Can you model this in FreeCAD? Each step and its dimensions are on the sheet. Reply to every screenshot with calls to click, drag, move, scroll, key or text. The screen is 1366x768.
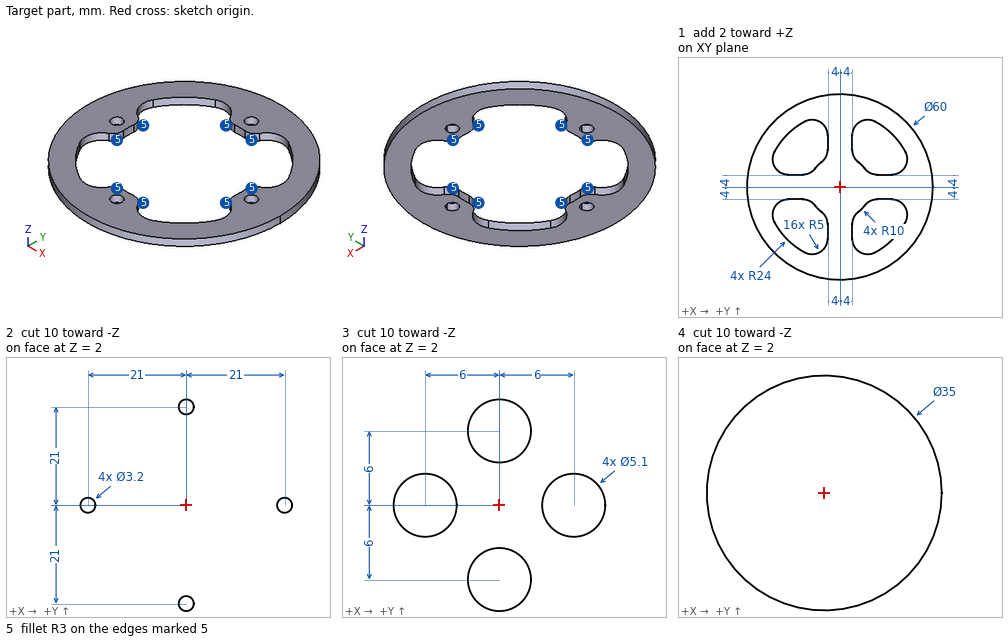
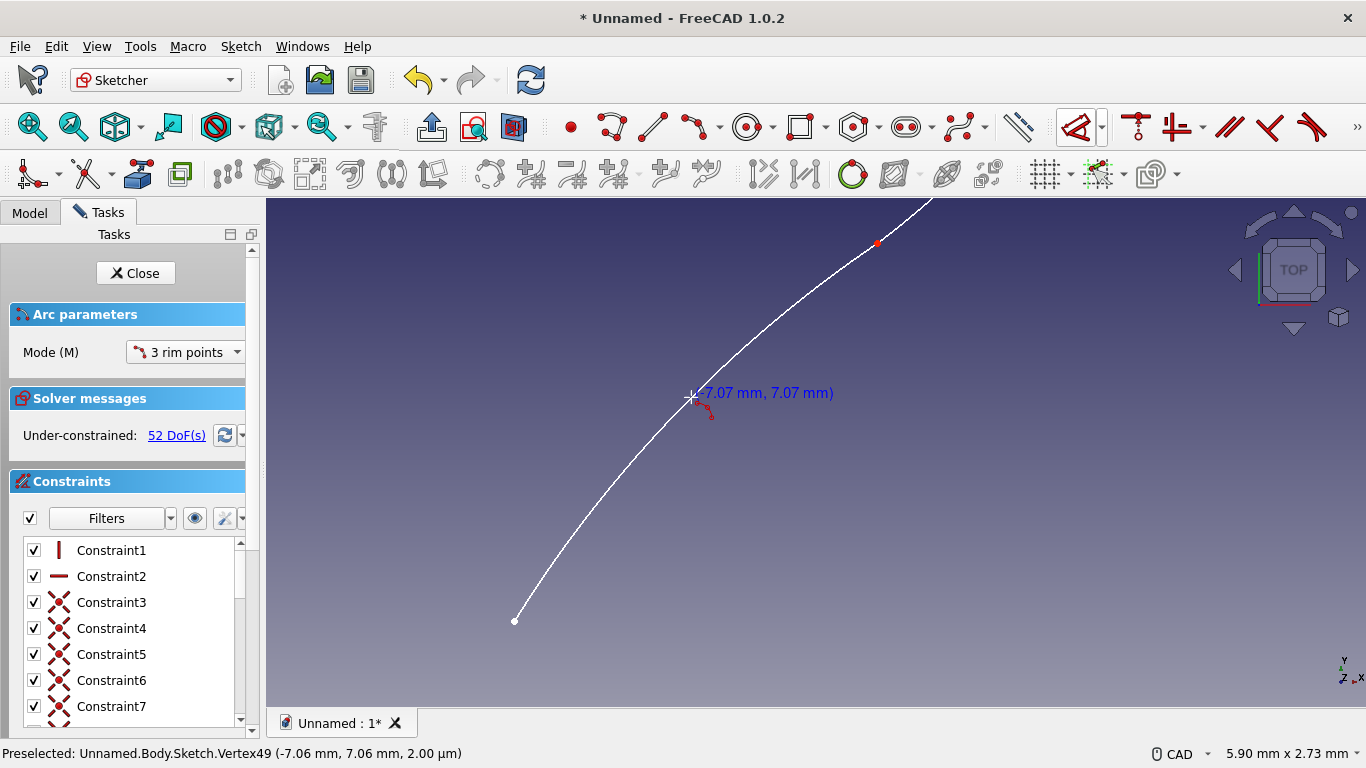
scroll(704, 409, down, 17)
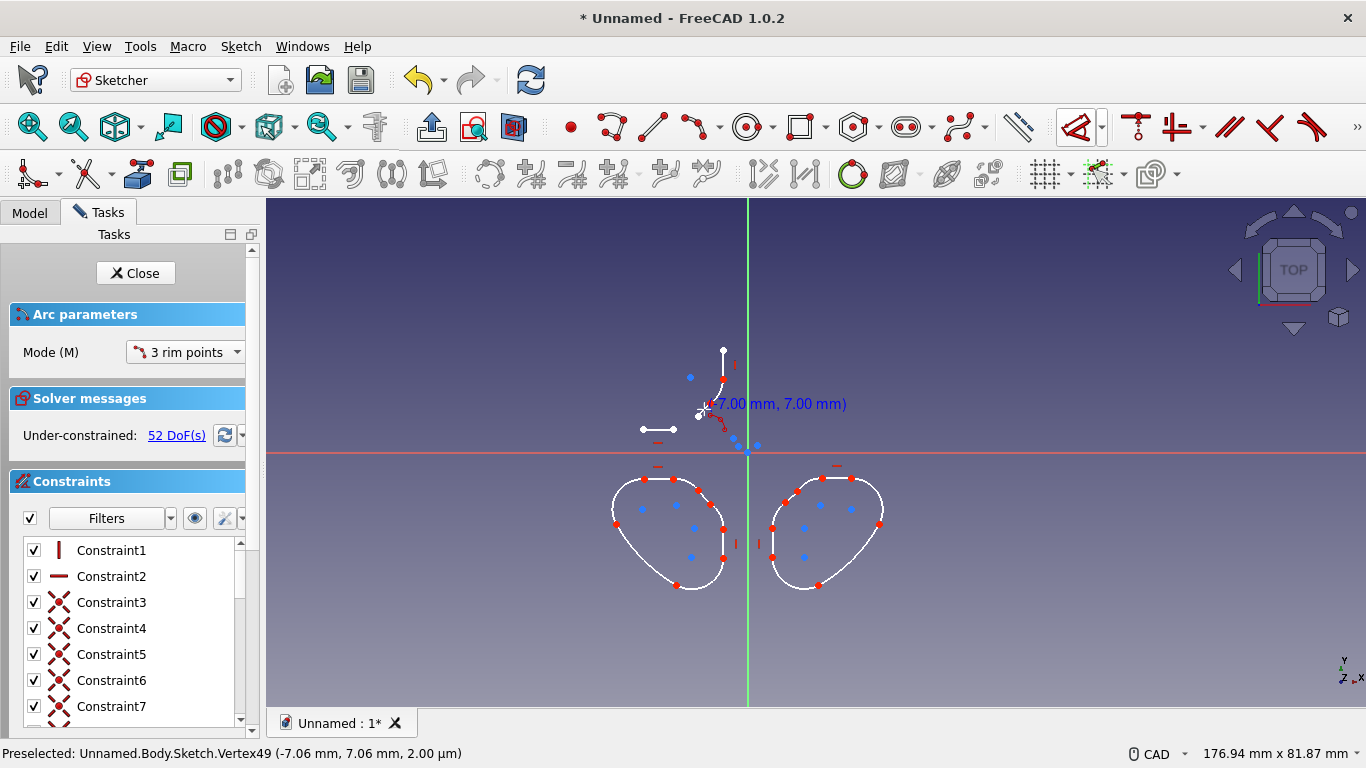
click(698, 416)
click(673, 430)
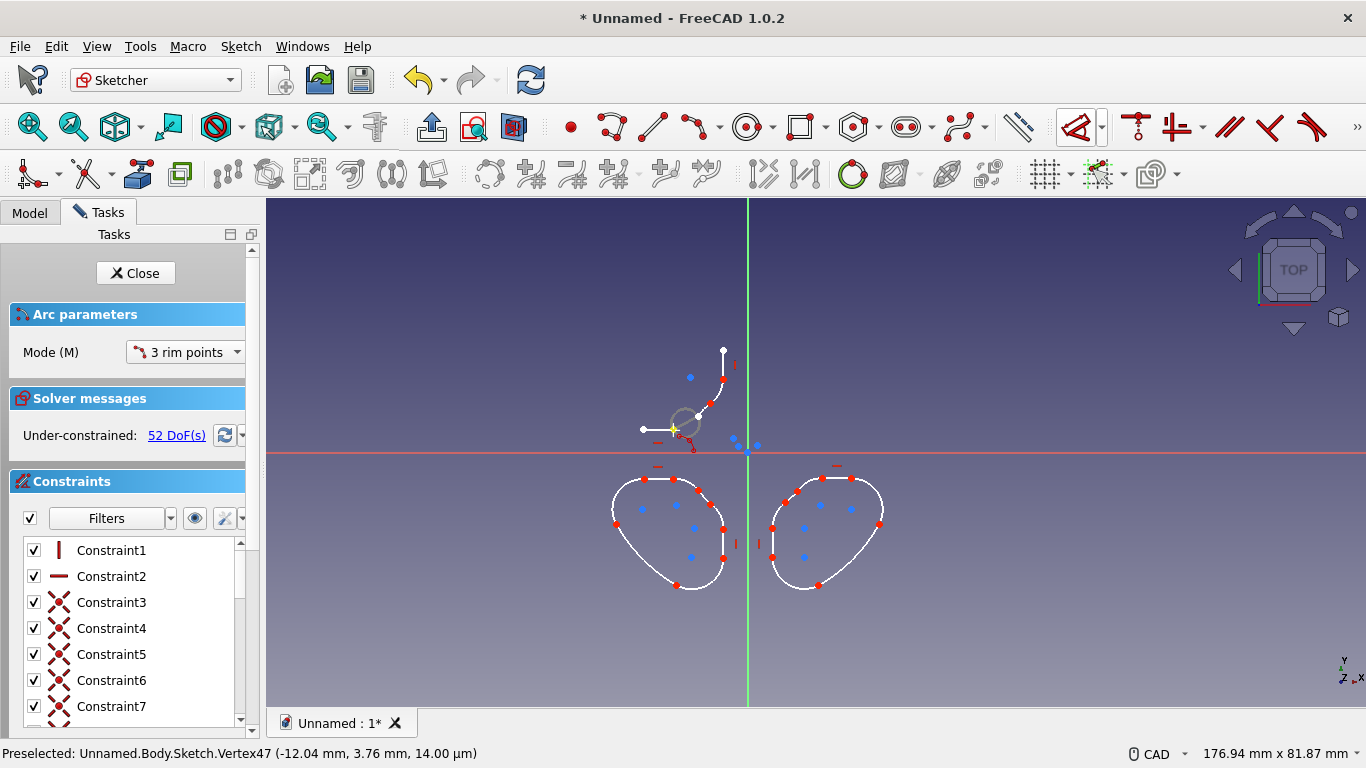
scroll(687, 425, up, 8)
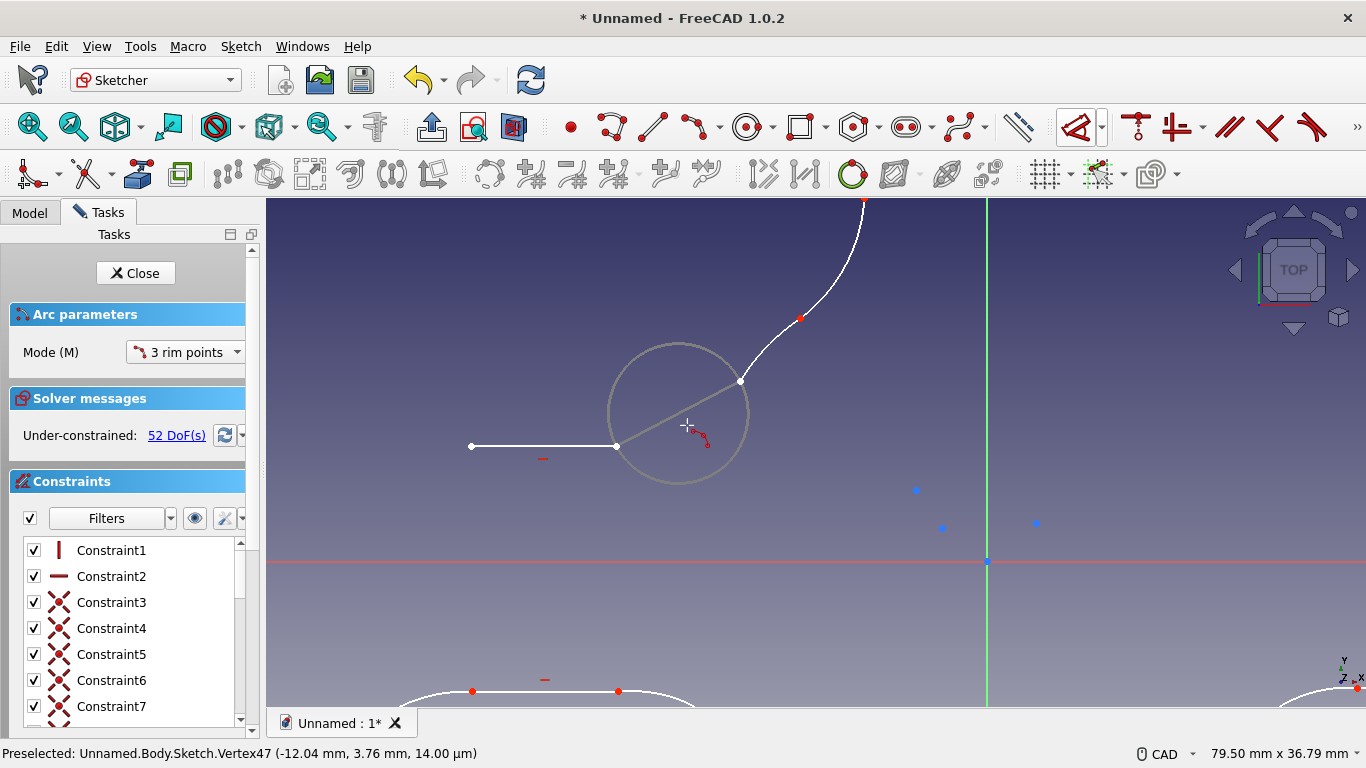
click(686, 422)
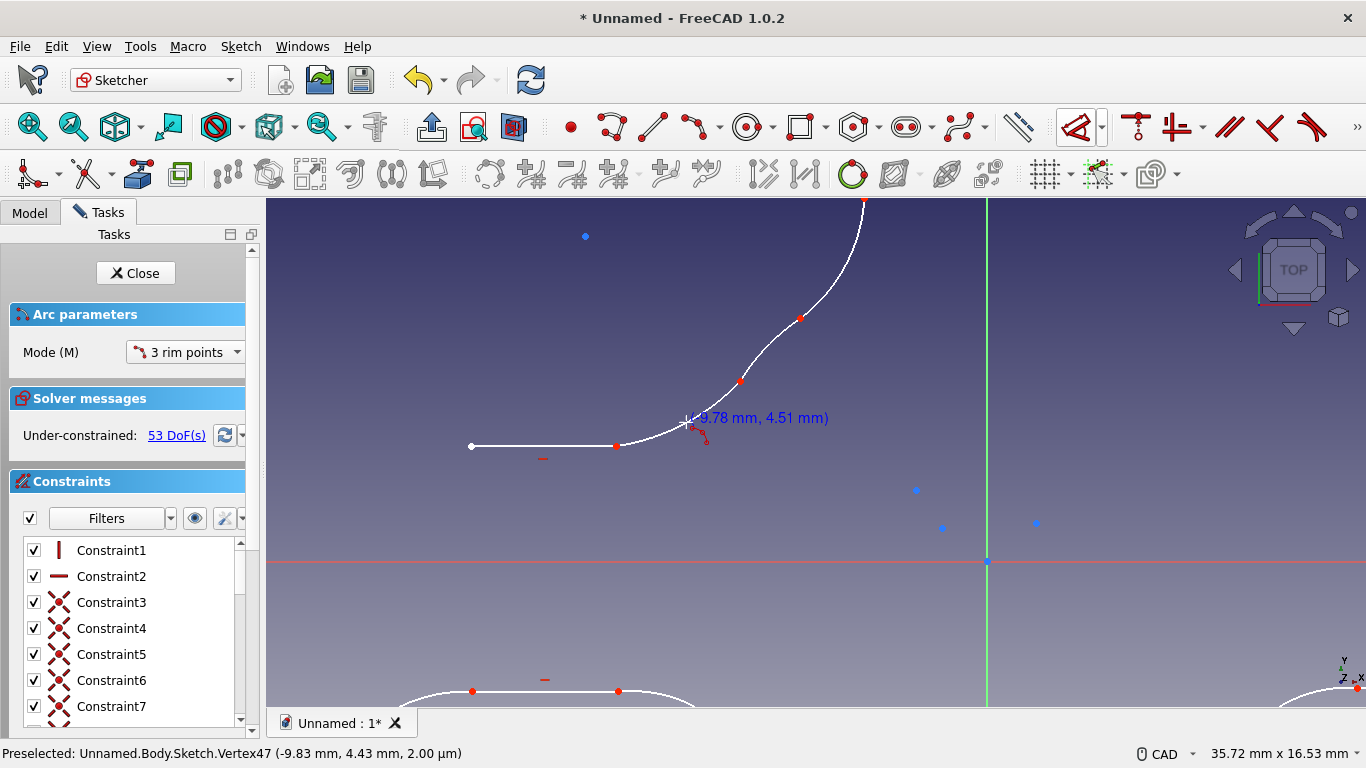
scroll(700, 431, down, 9)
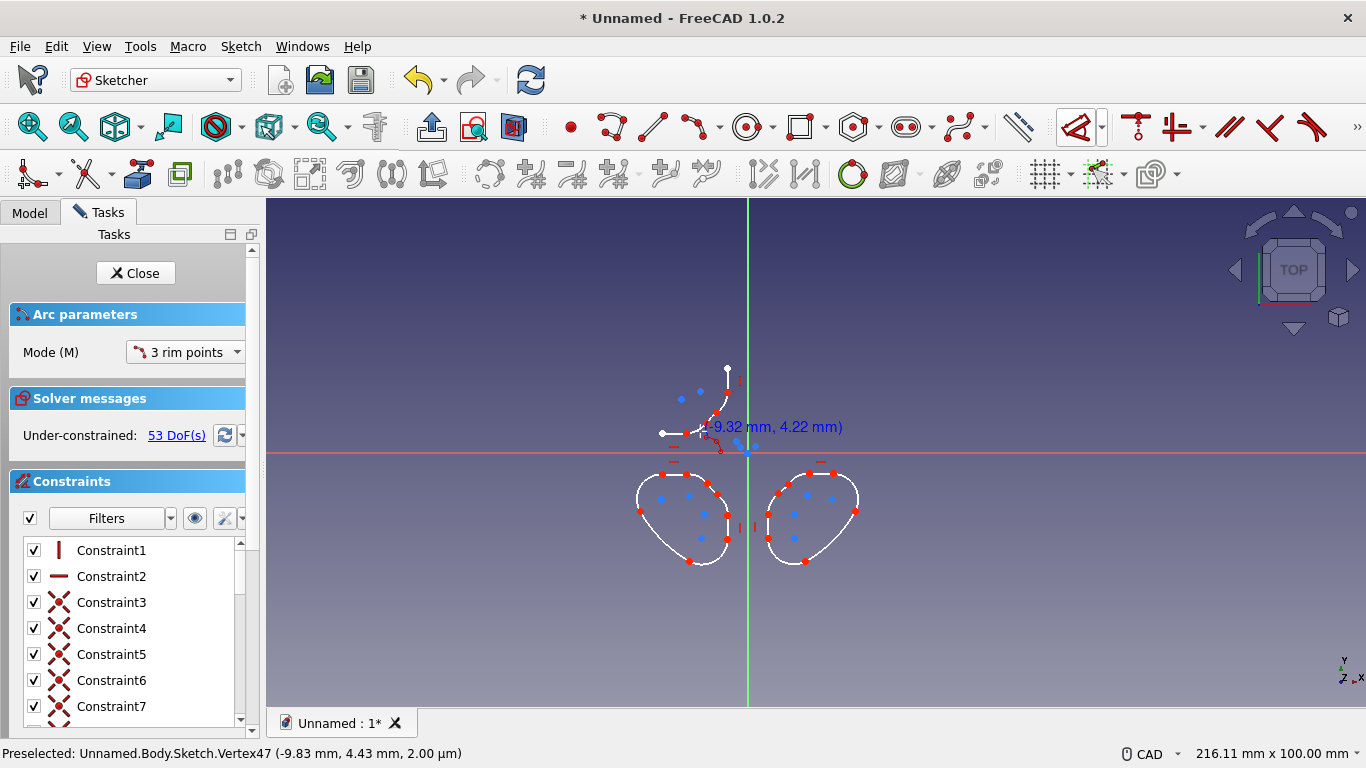
scroll(663, 433, up, 2)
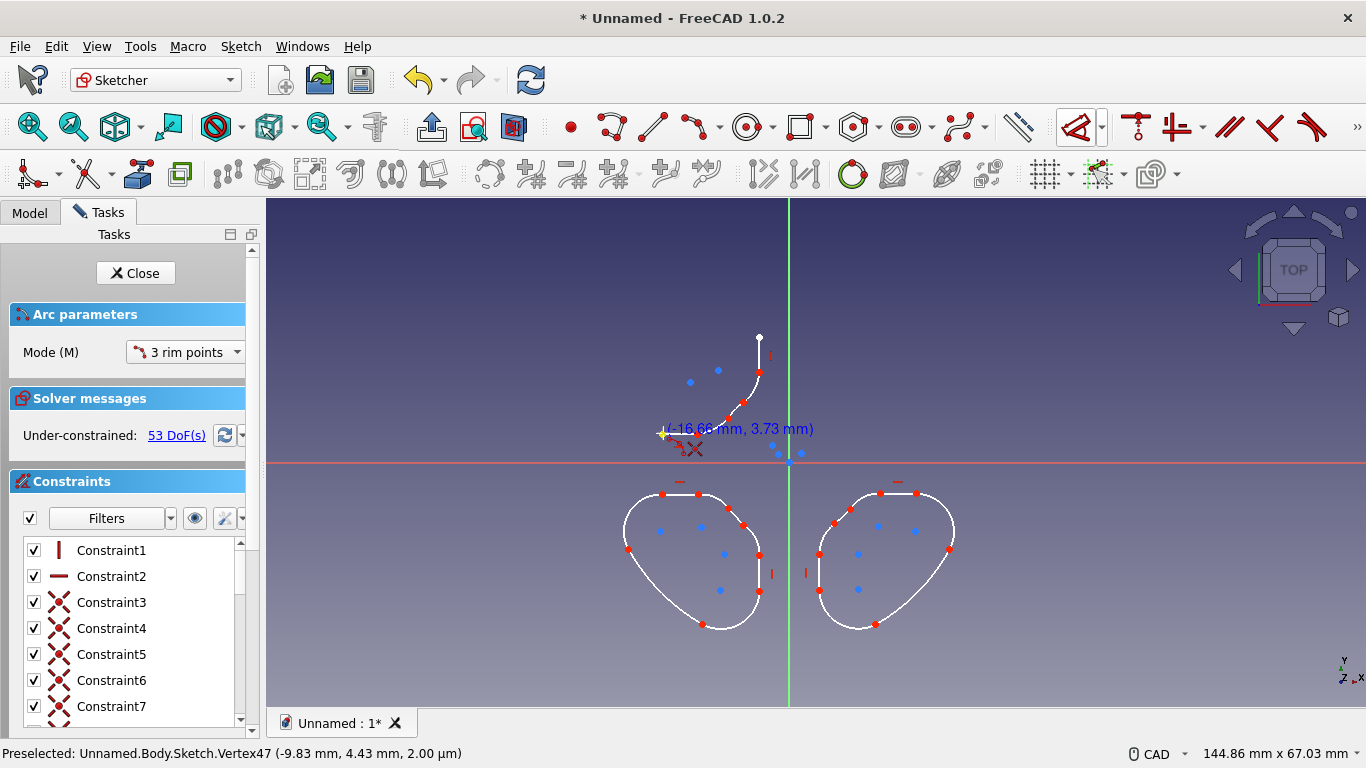
click(662, 434)
click(629, 376)
click(630, 414)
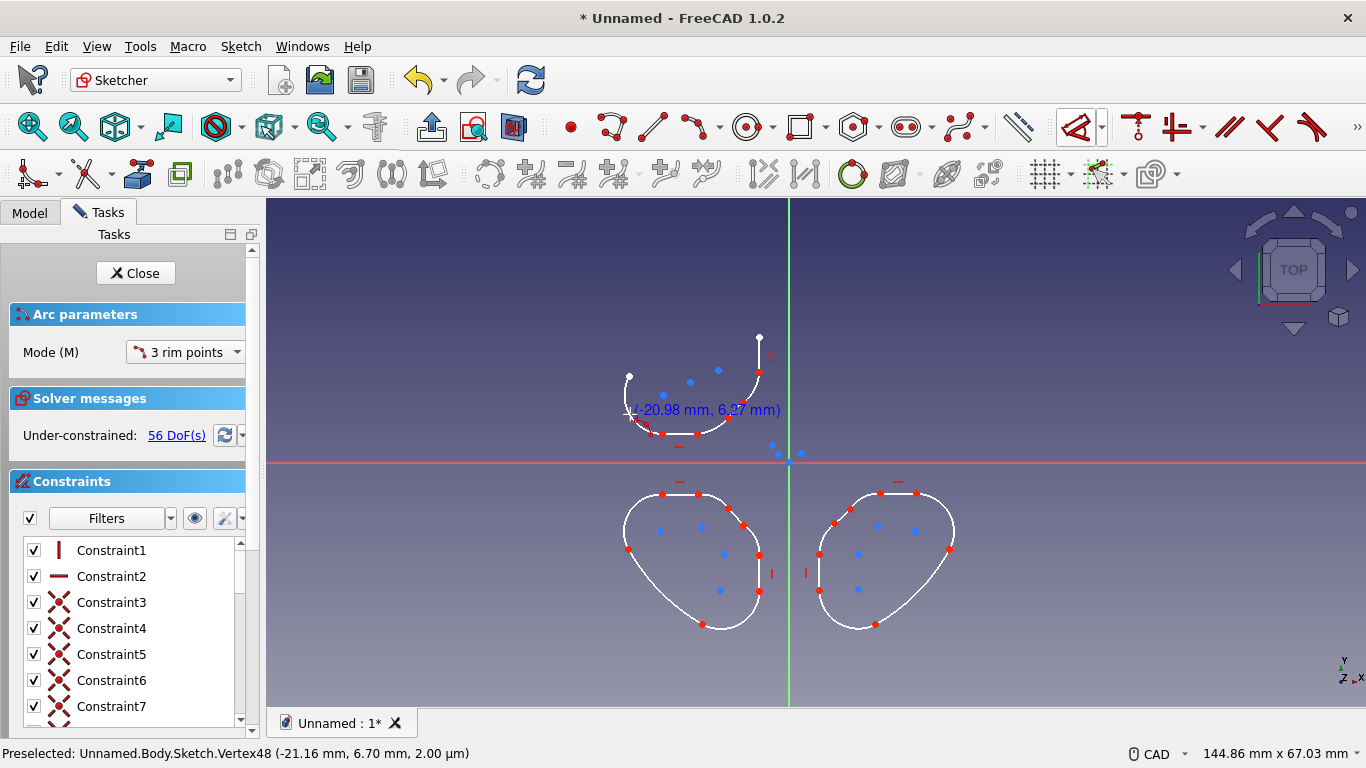
click(629, 377)
click(703, 302)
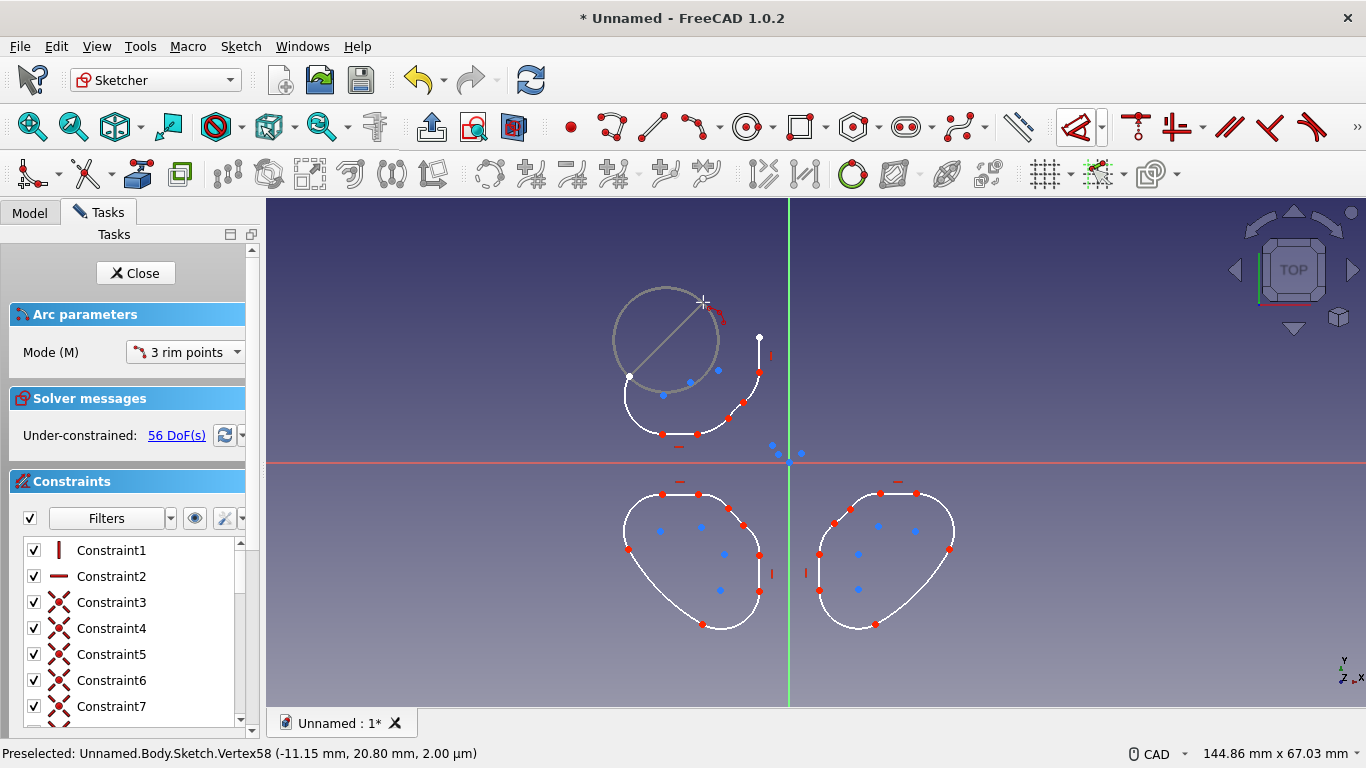
scroll(660, 334, up, 4)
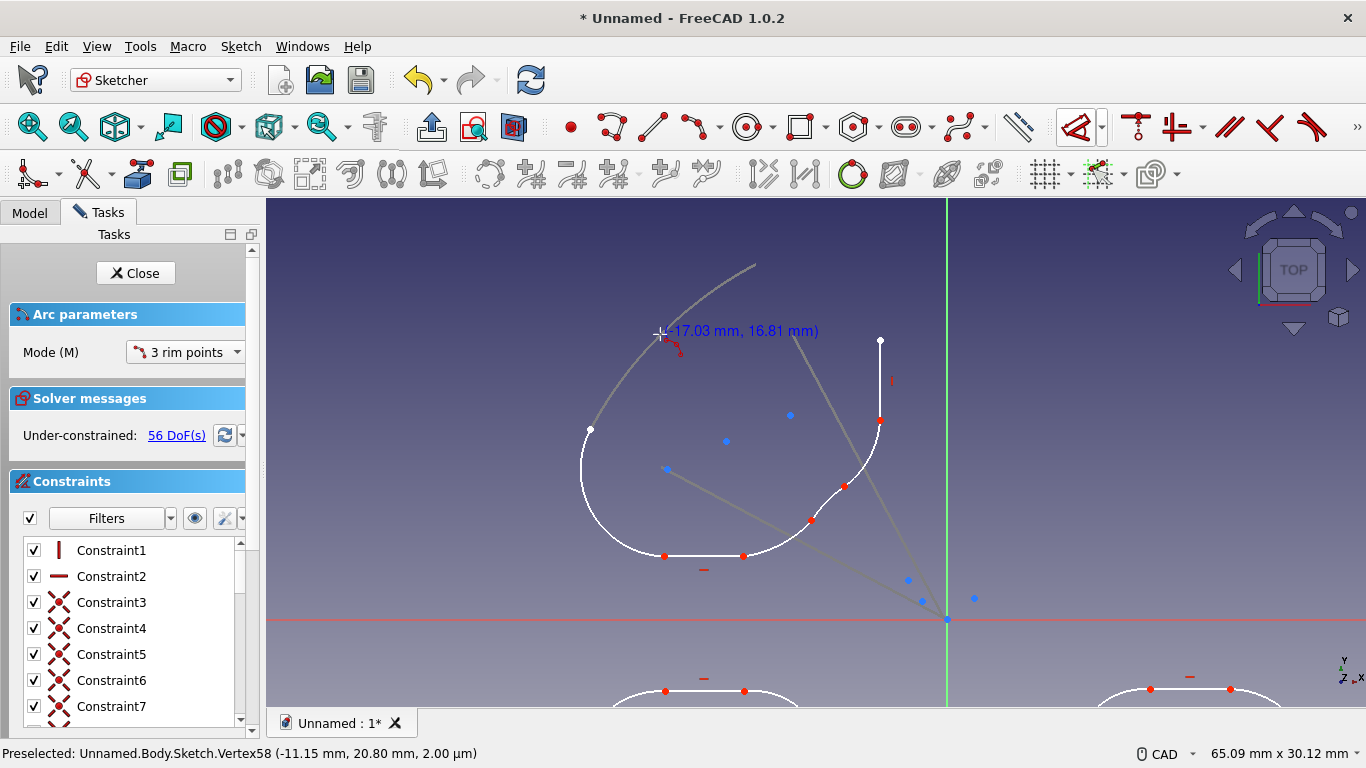
click(661, 333)